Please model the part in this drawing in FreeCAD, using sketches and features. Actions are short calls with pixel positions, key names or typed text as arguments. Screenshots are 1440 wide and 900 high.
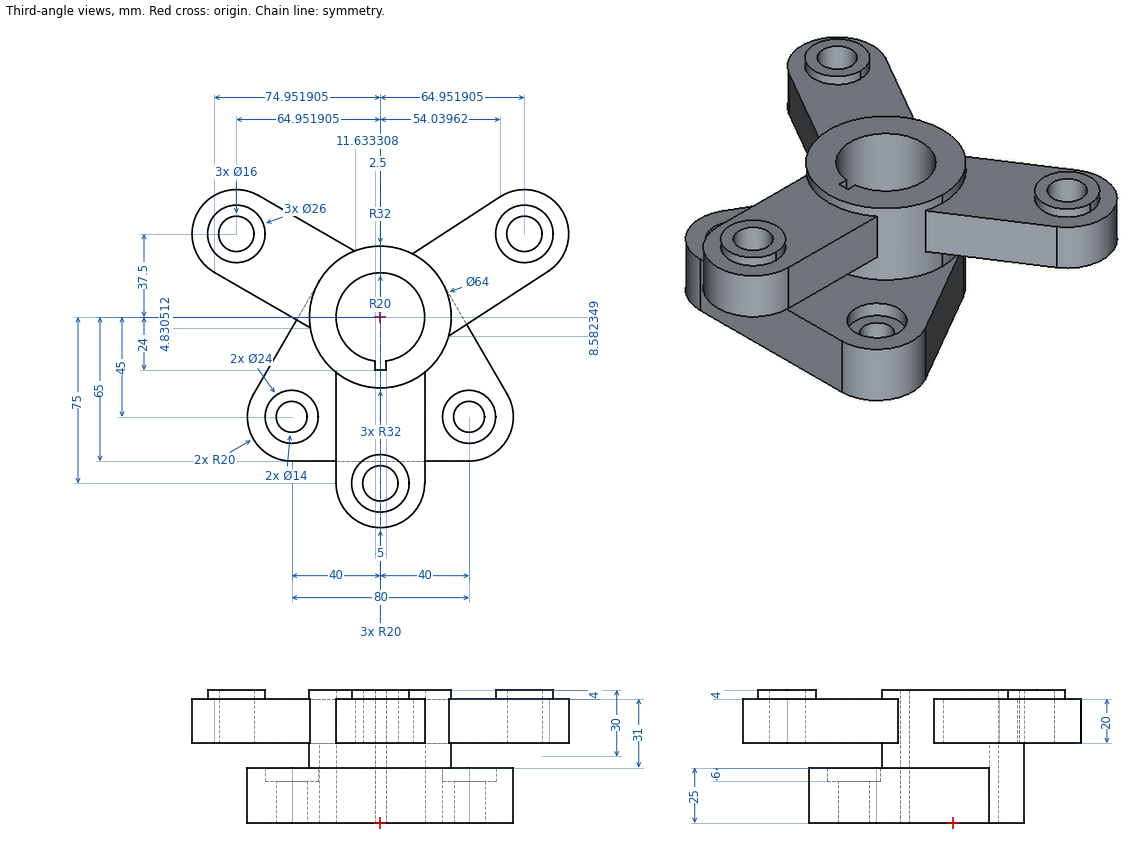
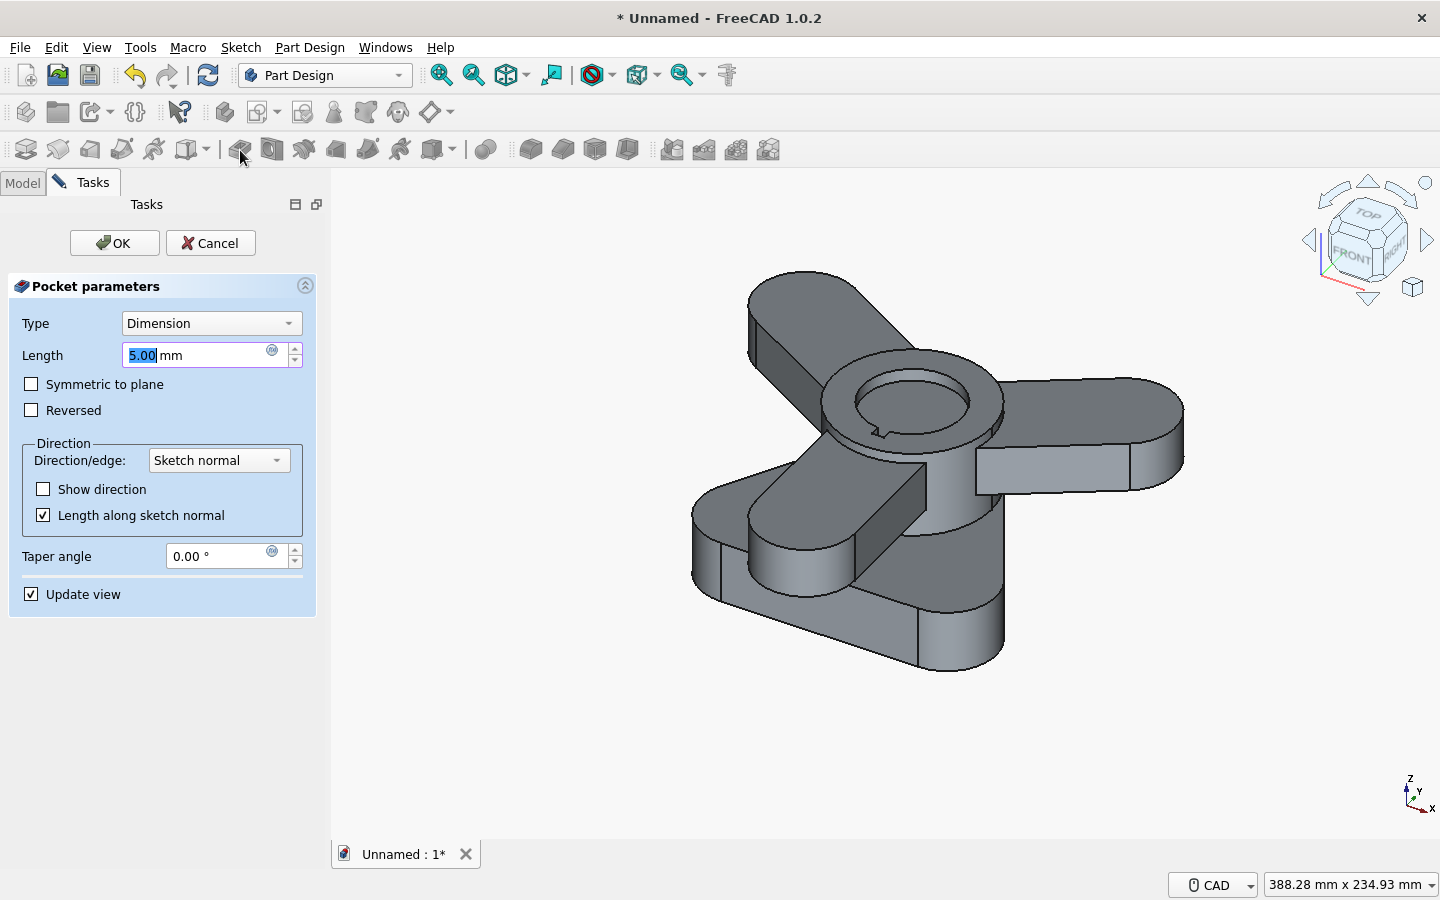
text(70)
key(Tab)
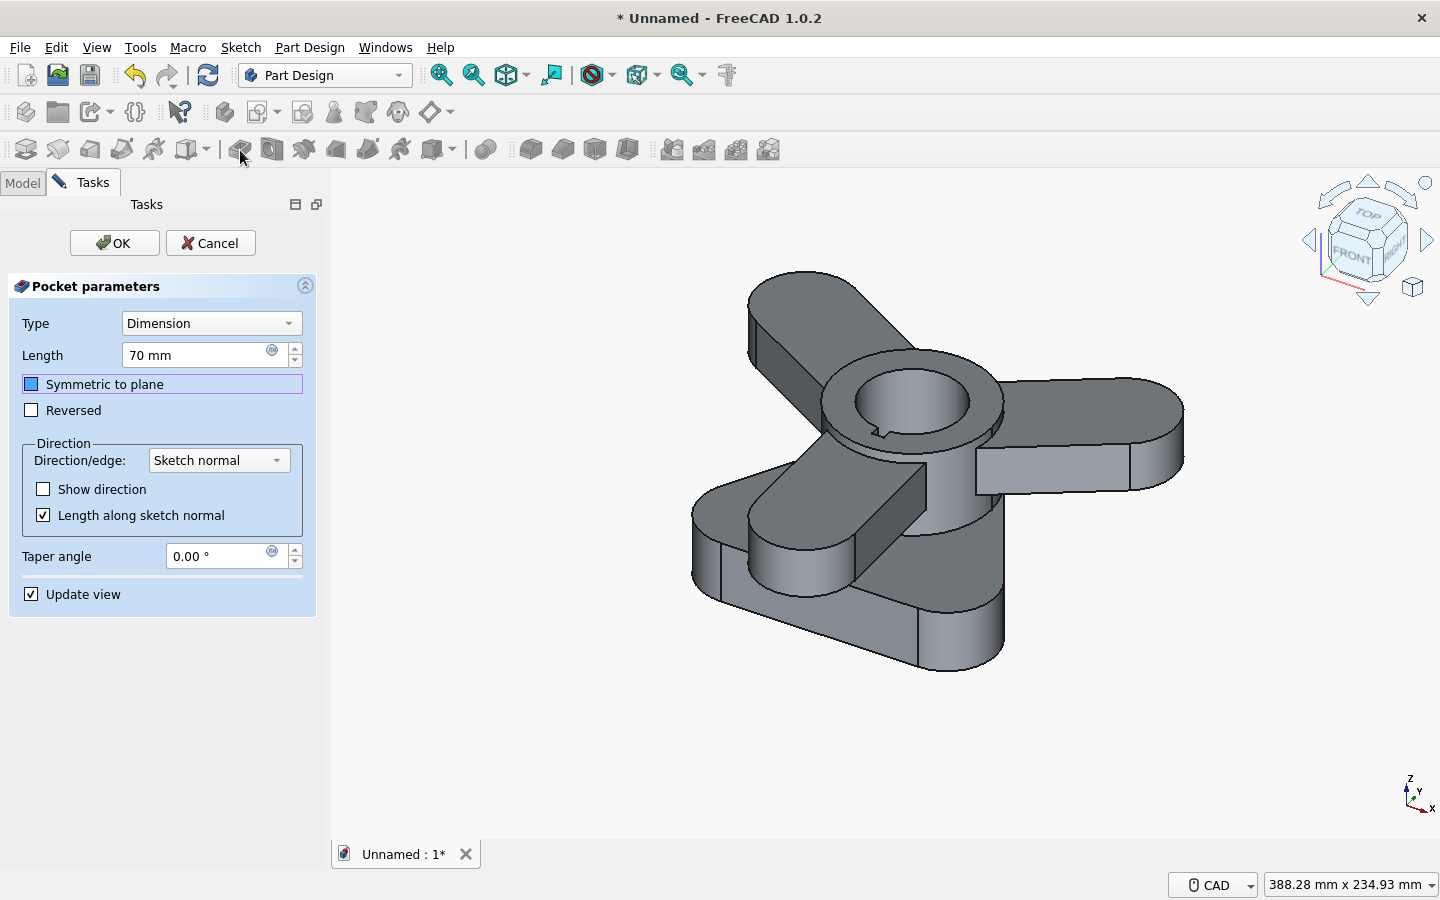
click(115, 243)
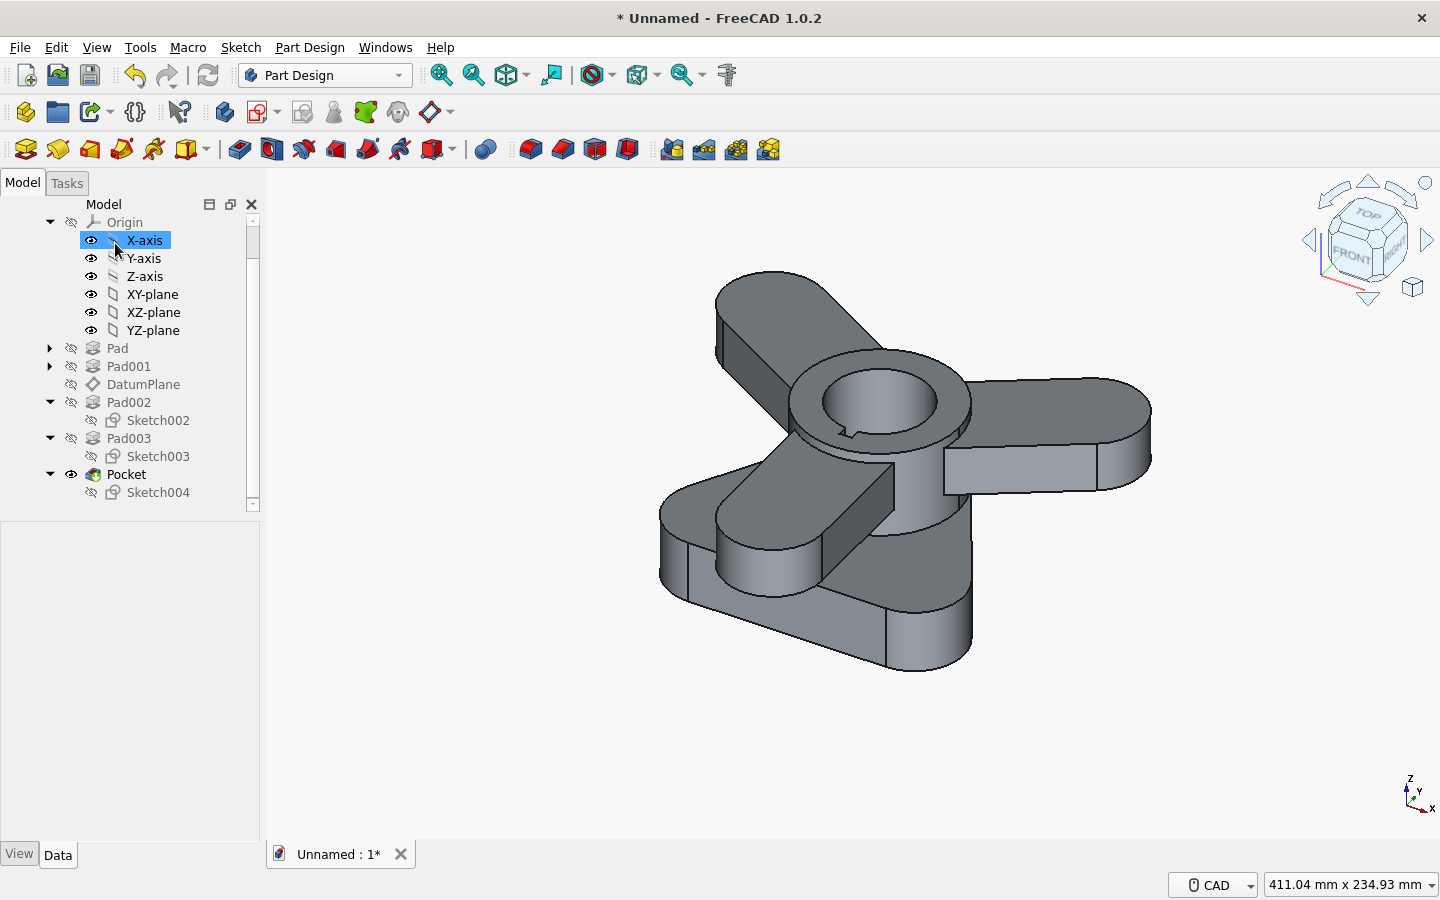
click(1076, 411)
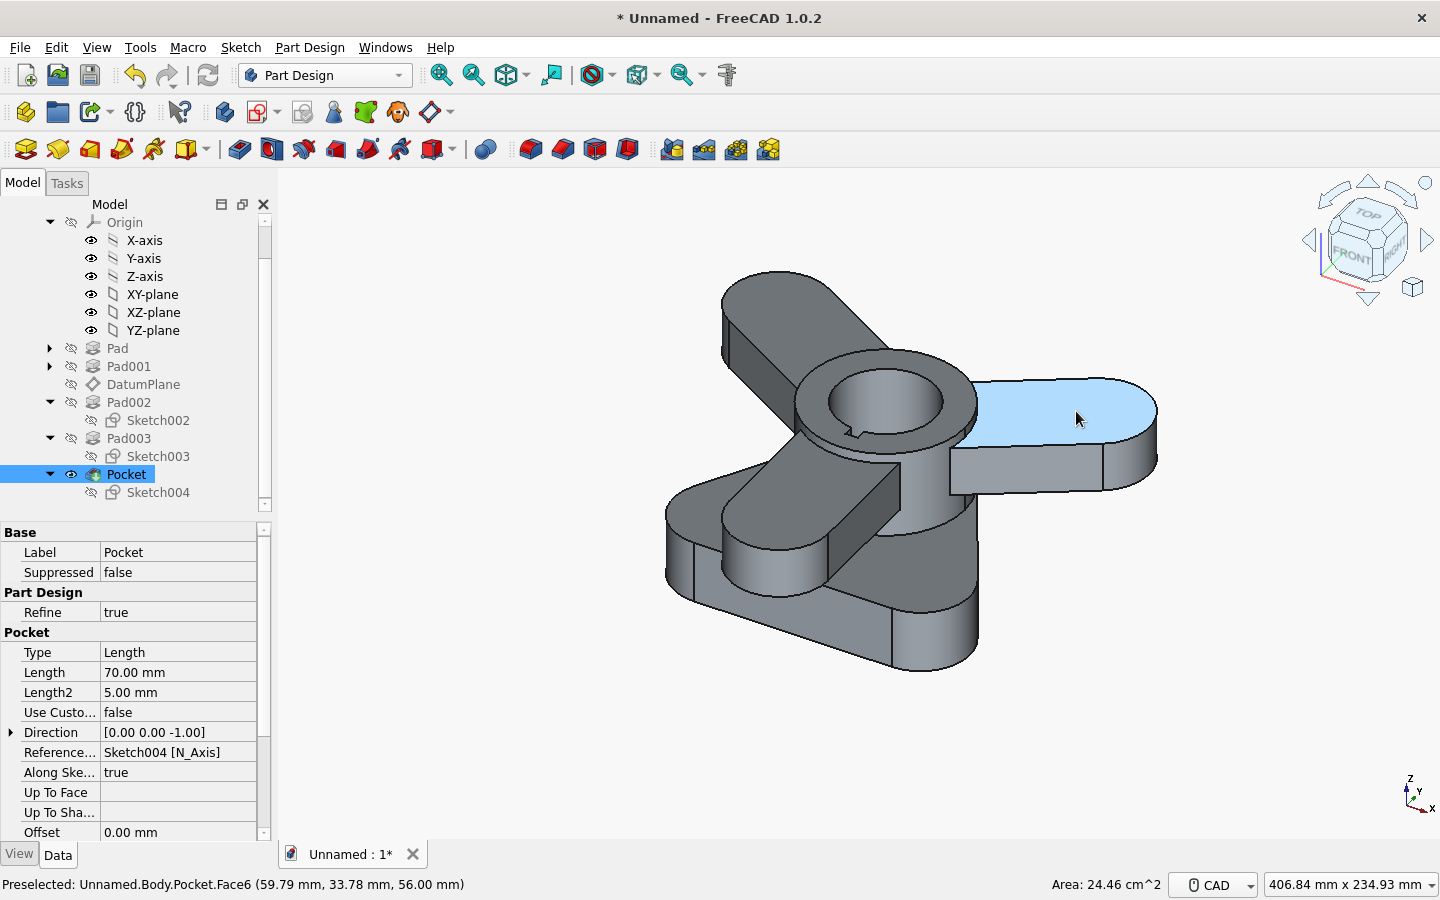
click(258, 112)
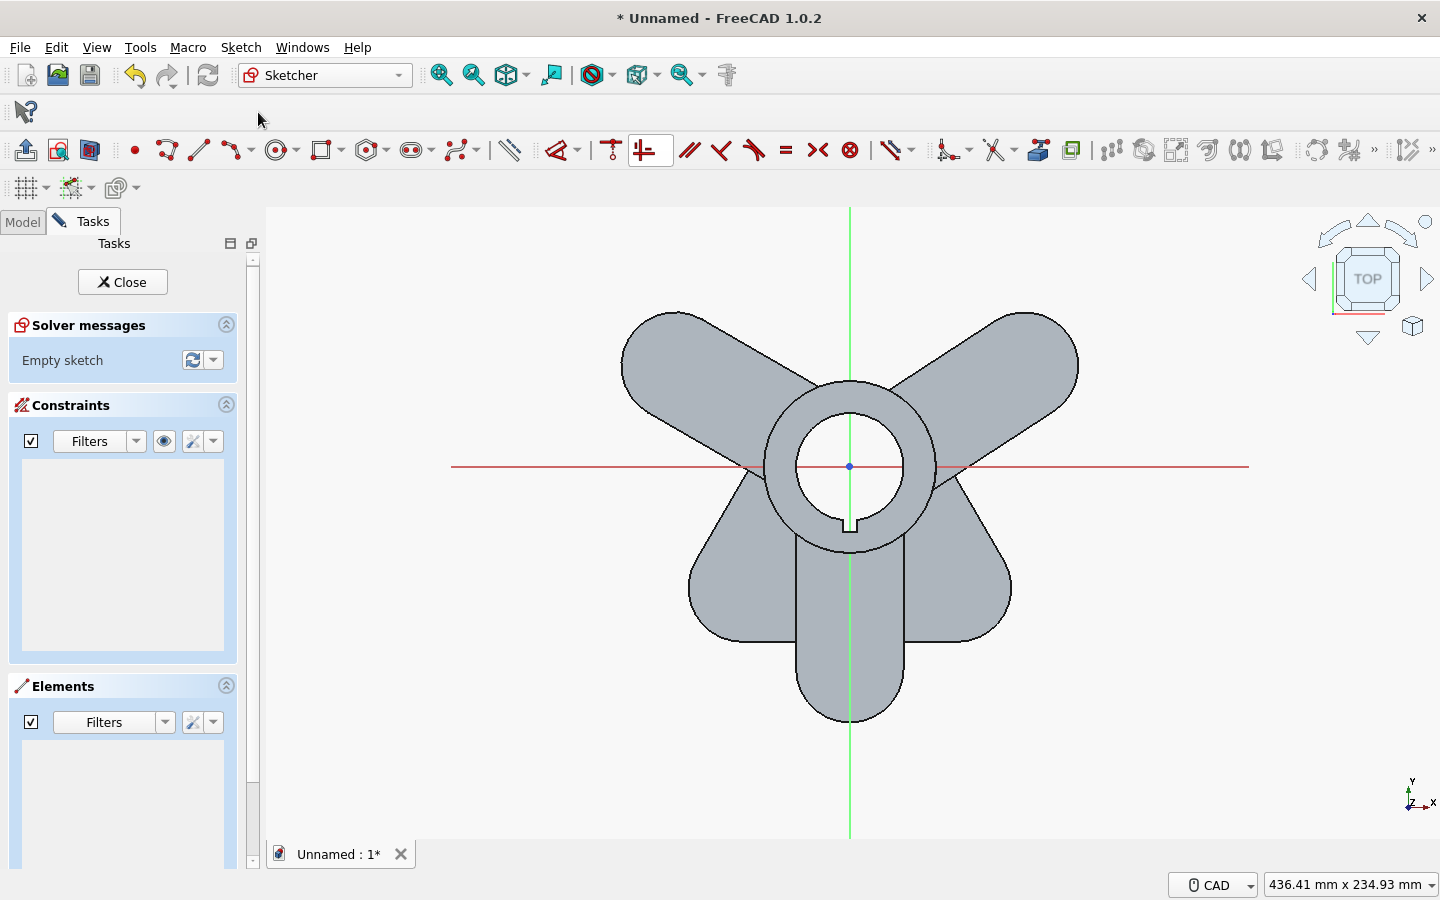
click(90, 150)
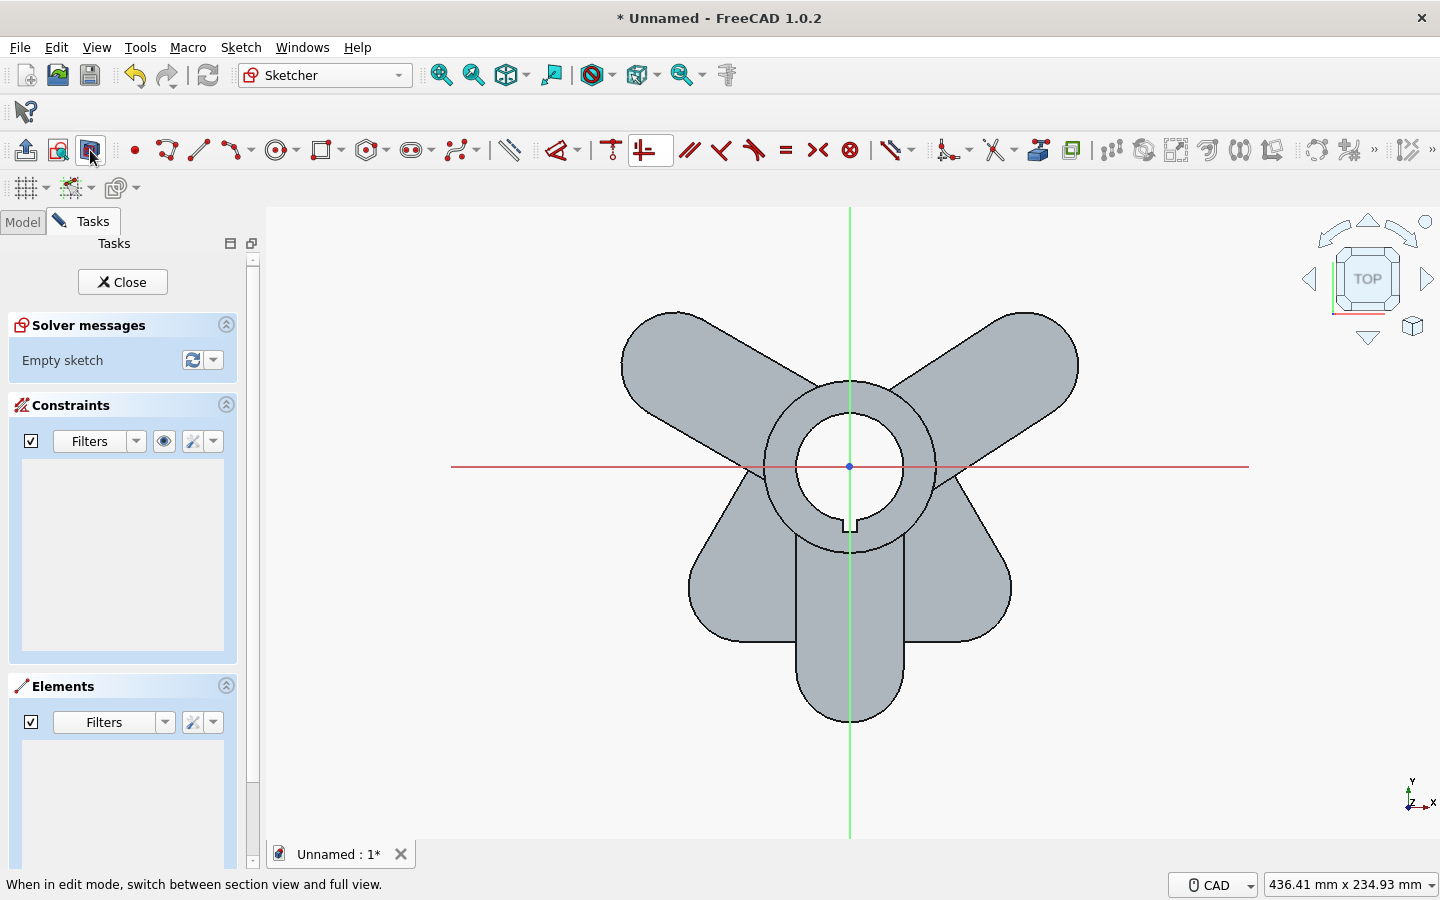
click(276, 150)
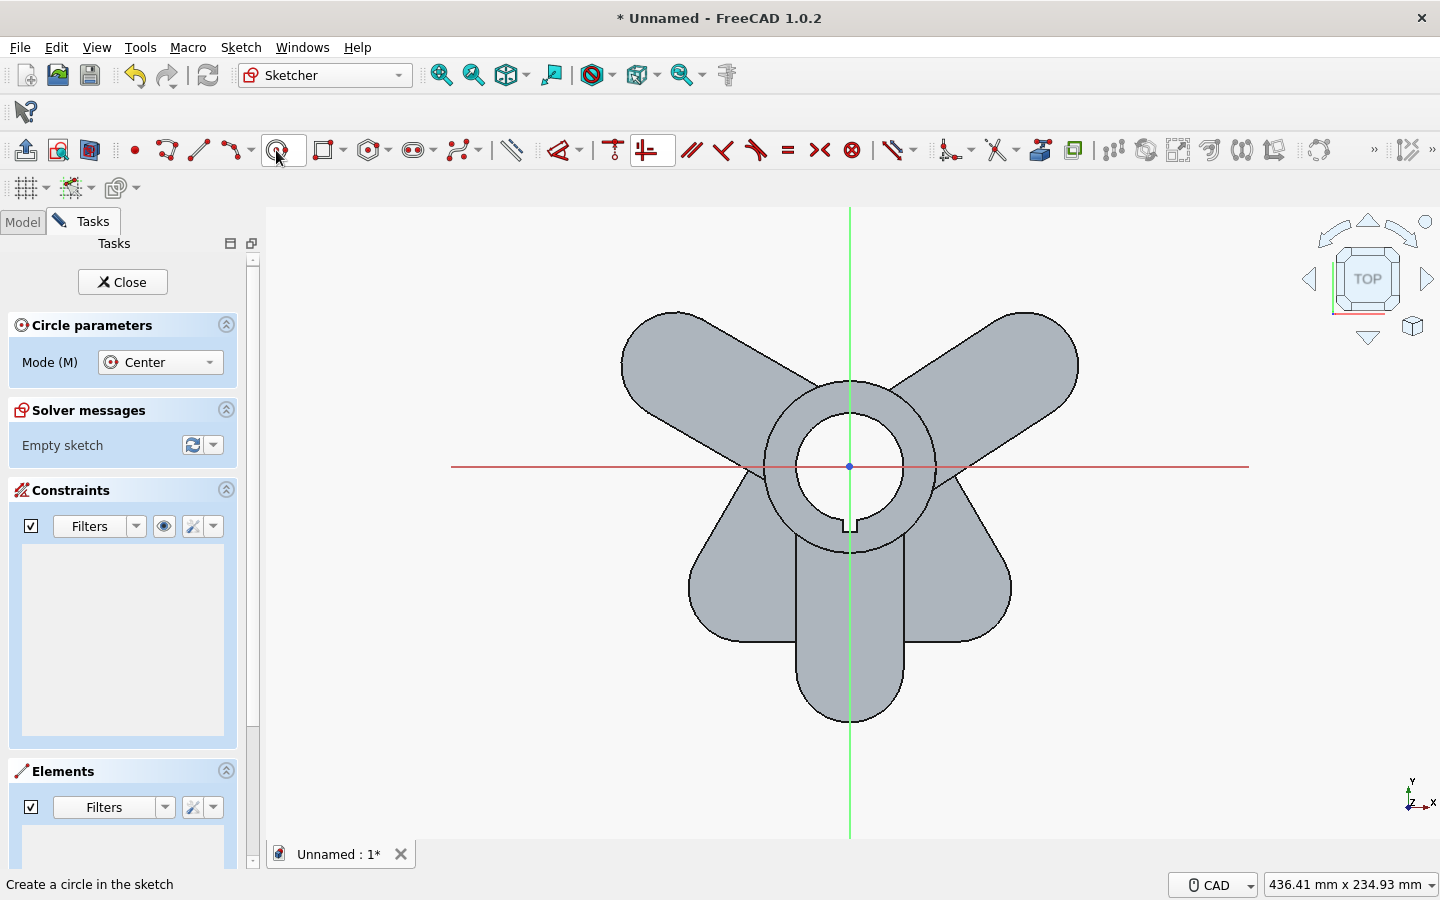
click(675, 366)
move(700, 341)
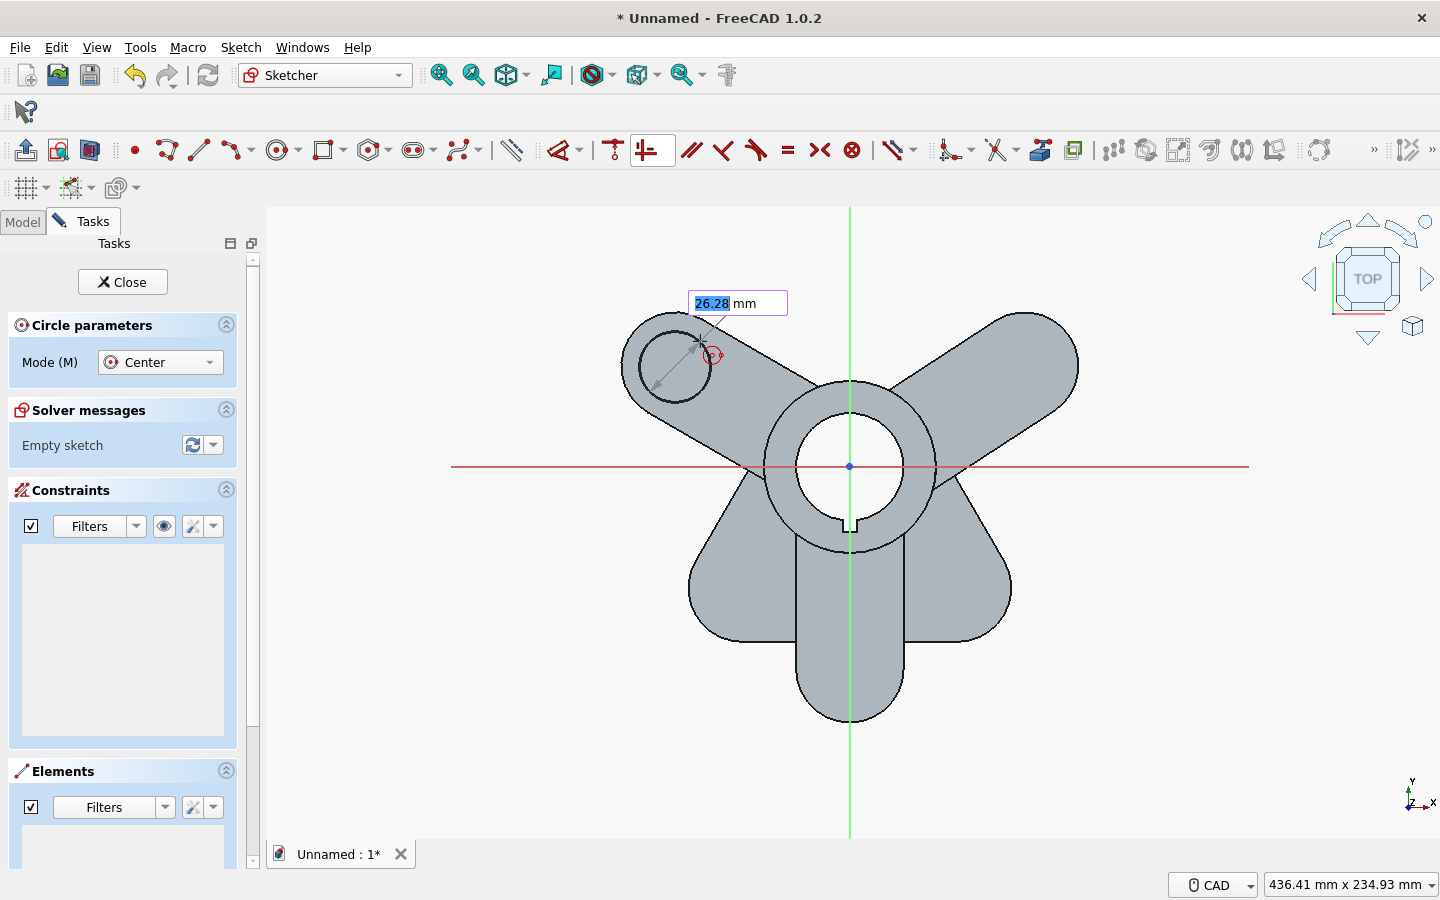
text(26)
key(Return)